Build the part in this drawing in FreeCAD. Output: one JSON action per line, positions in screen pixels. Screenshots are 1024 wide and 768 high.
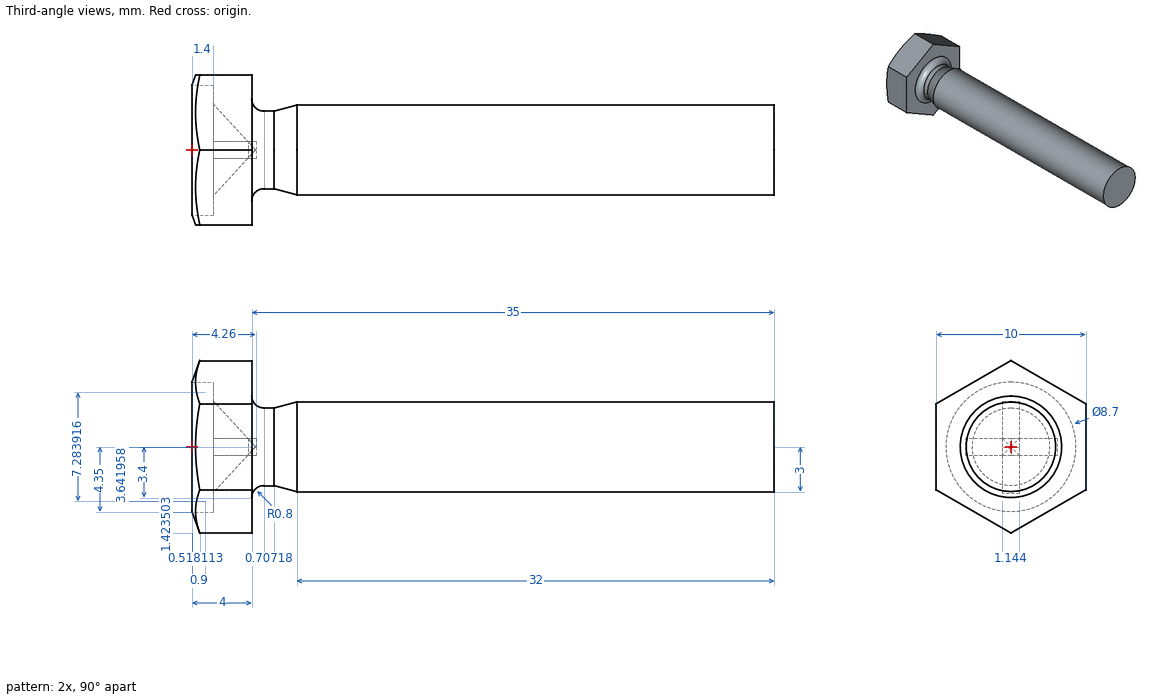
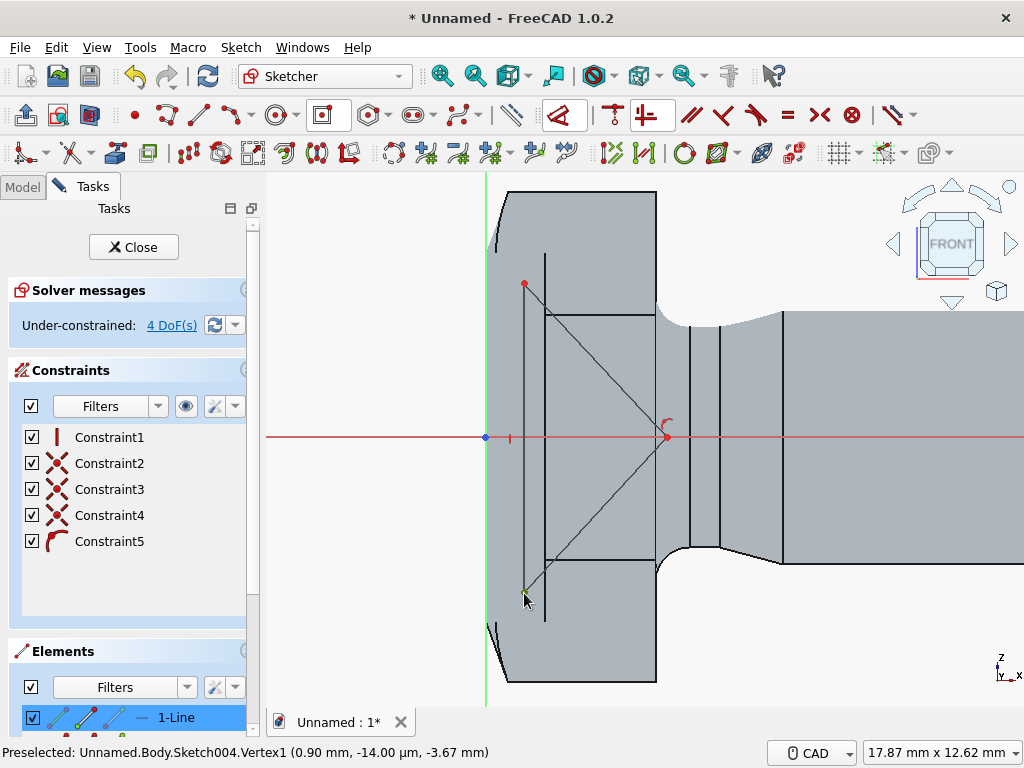
{"action": "left_click", "coordinate": [582, 116]}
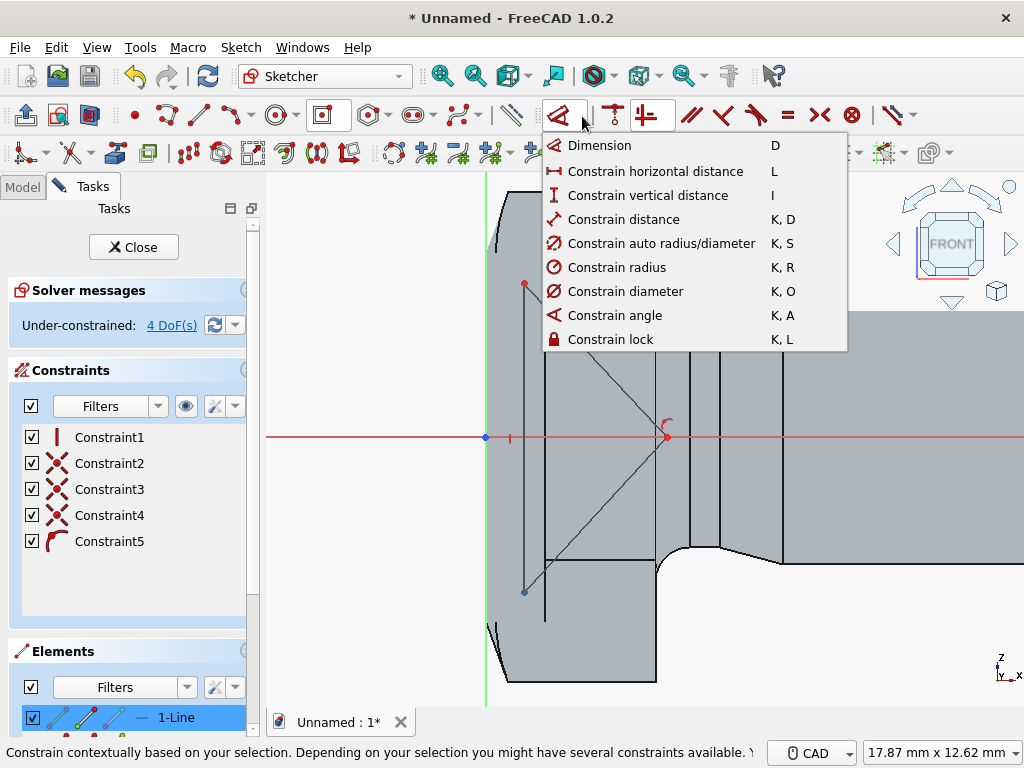
{"action": "left_click", "coordinate": [695, 171]}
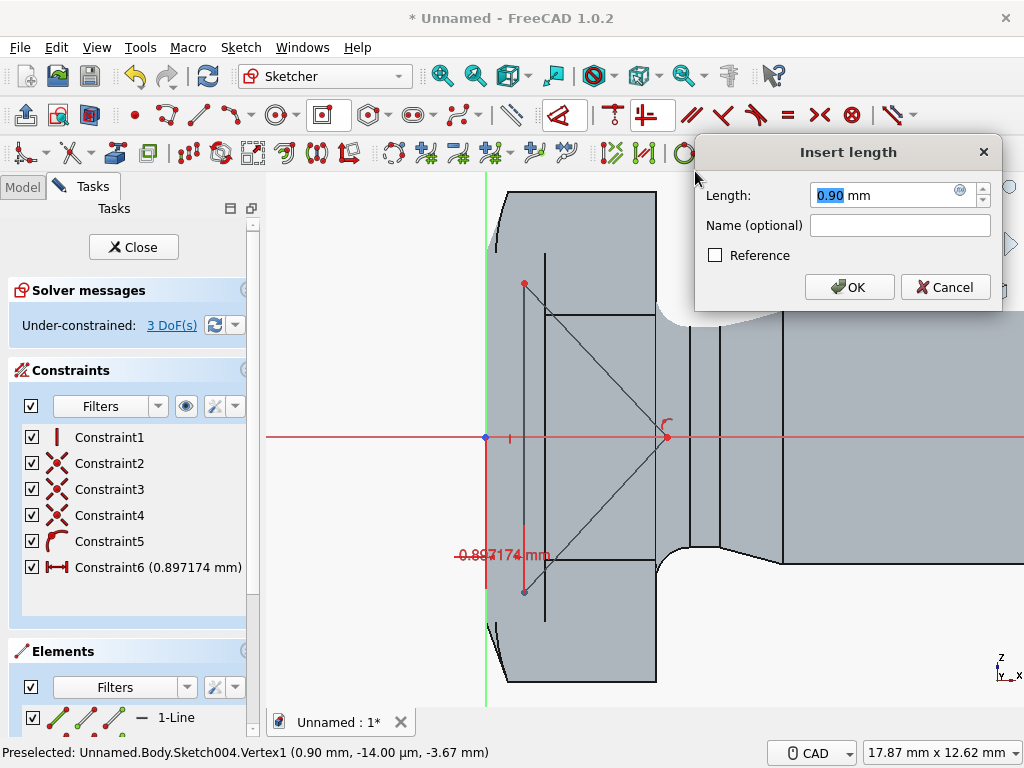
{"action": "type", "text": "0.9"}
{"action": "key", "text": "Return"}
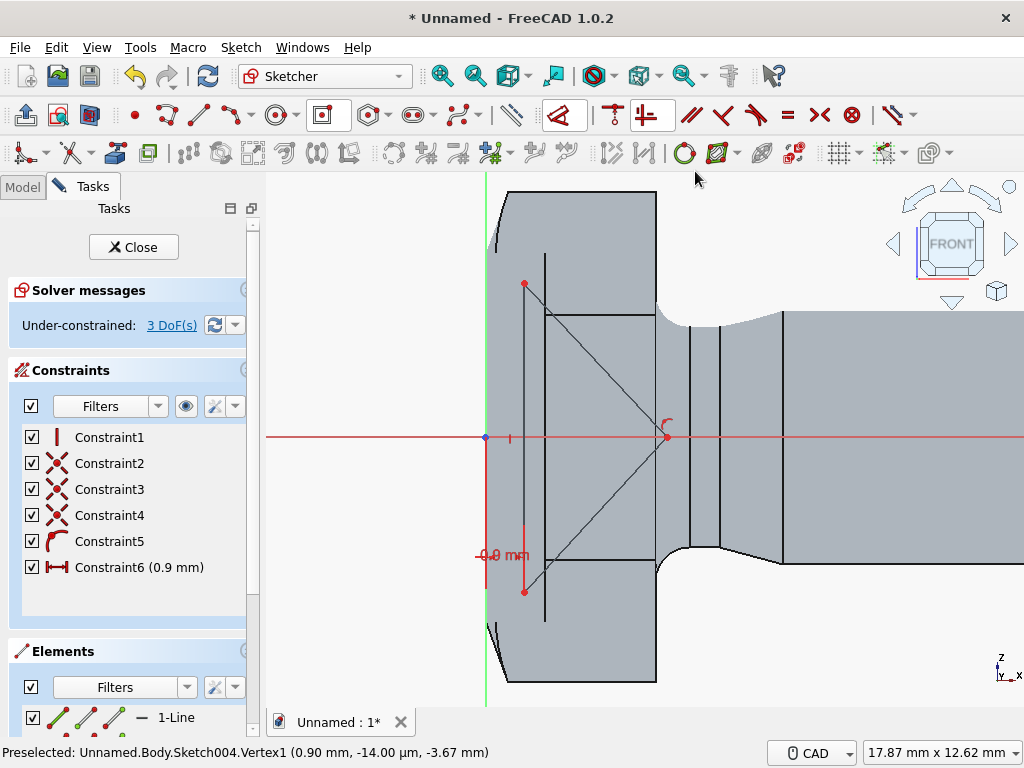
{"action": "left_click", "coordinate": [667, 437]}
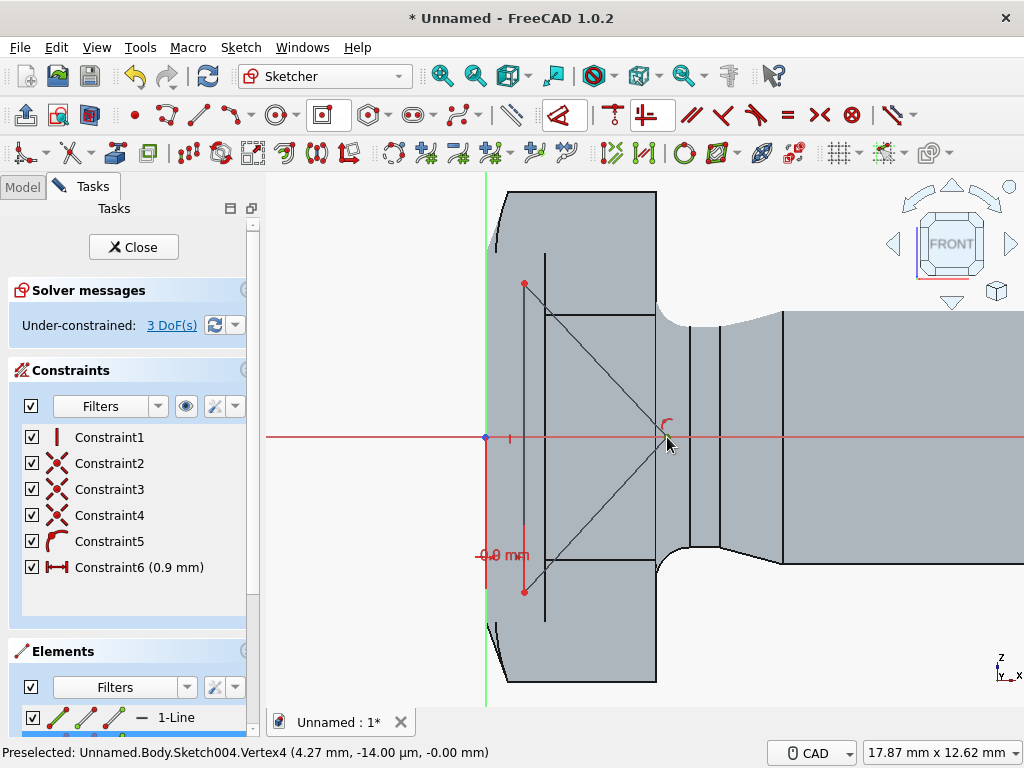
{"action": "key", "text": "l"}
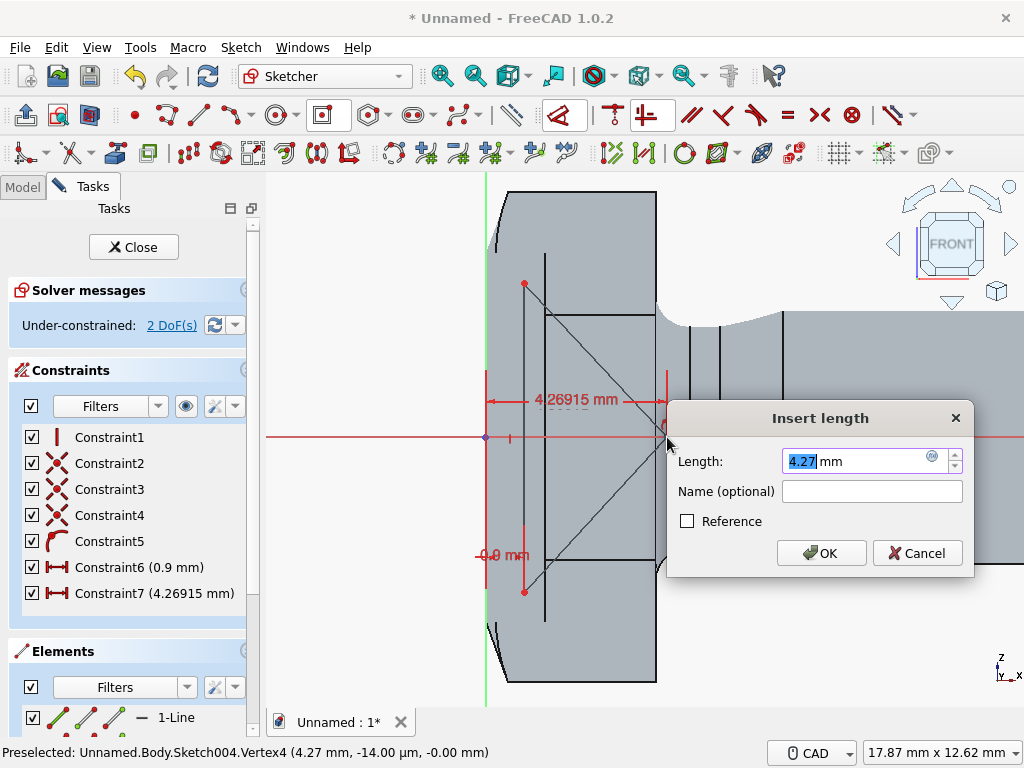
{"action": "type", "text": "4.26"}
{"action": "key", "text": "Return"}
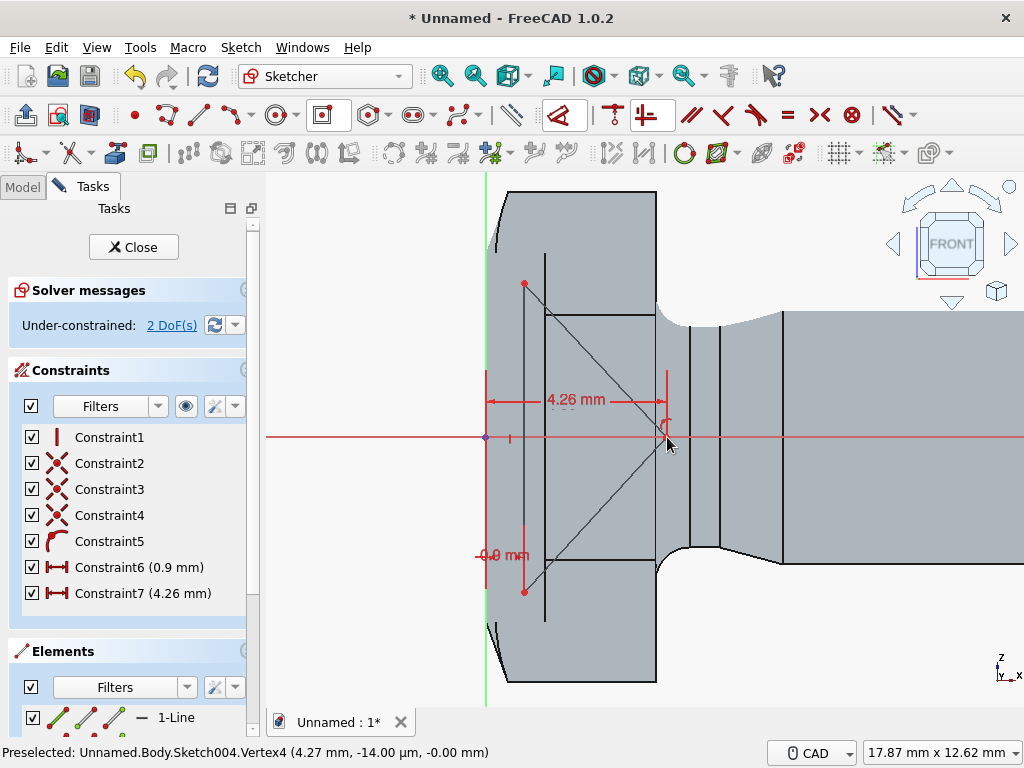
{"action": "left_click", "coordinate": [524, 500]}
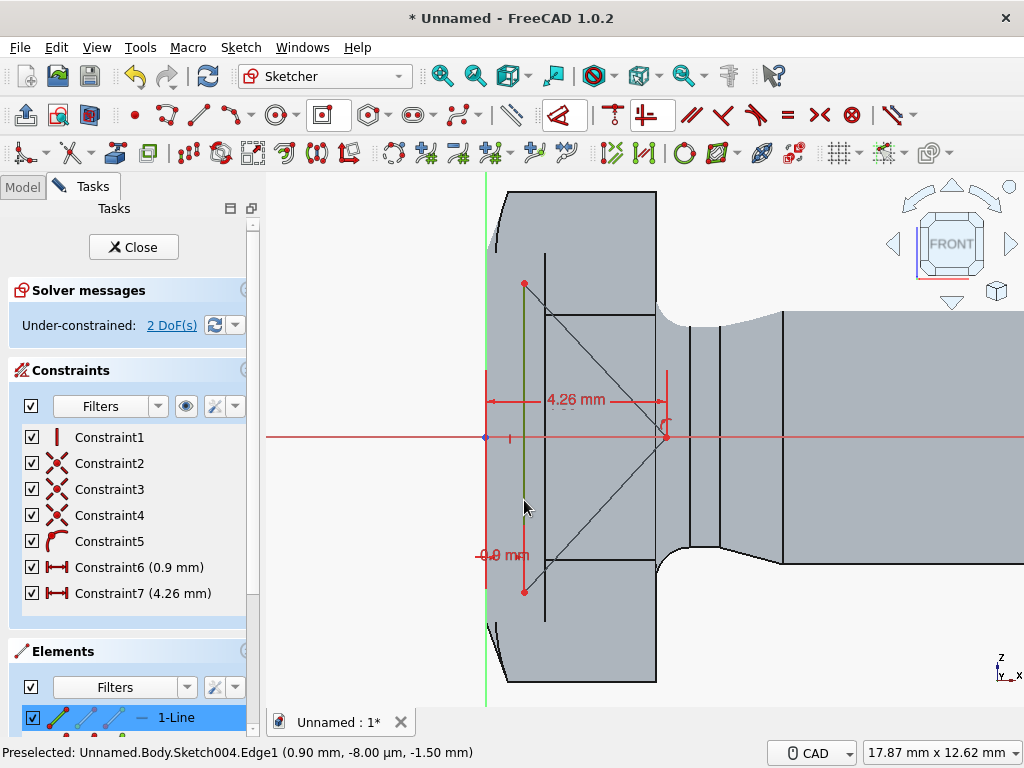
{"action": "key", "text": "i"}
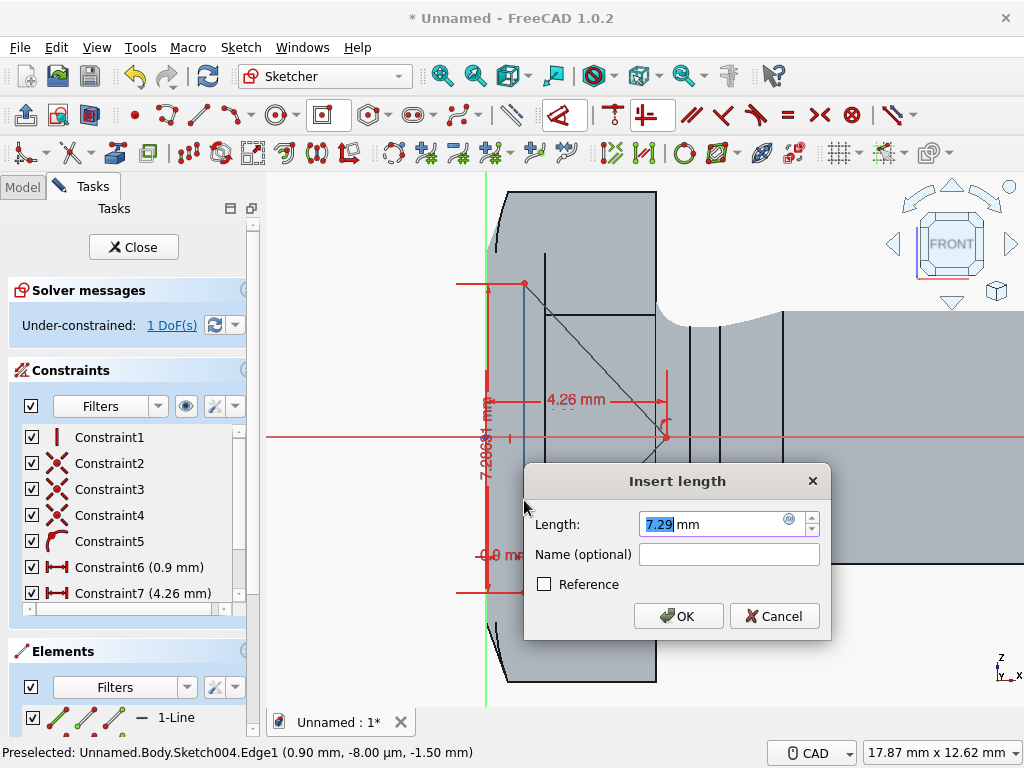
{"action": "type", "text": "7.283916"}
{"action": "key", "text": "Return"}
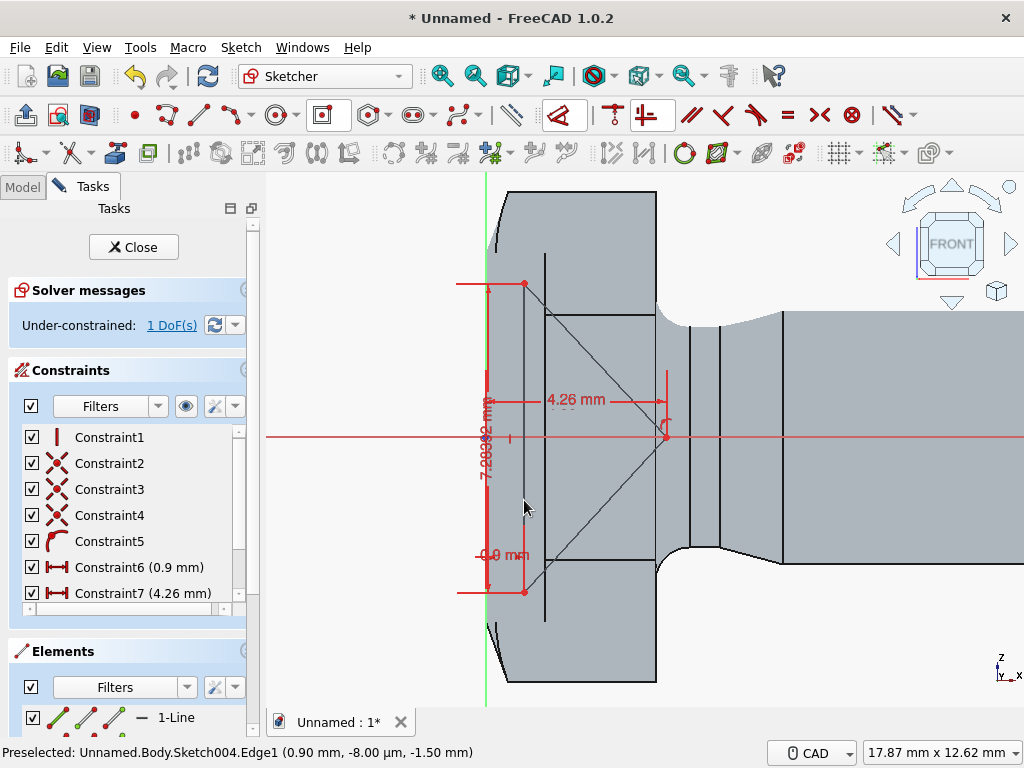
{"action": "left_click", "coordinate": [524, 593]}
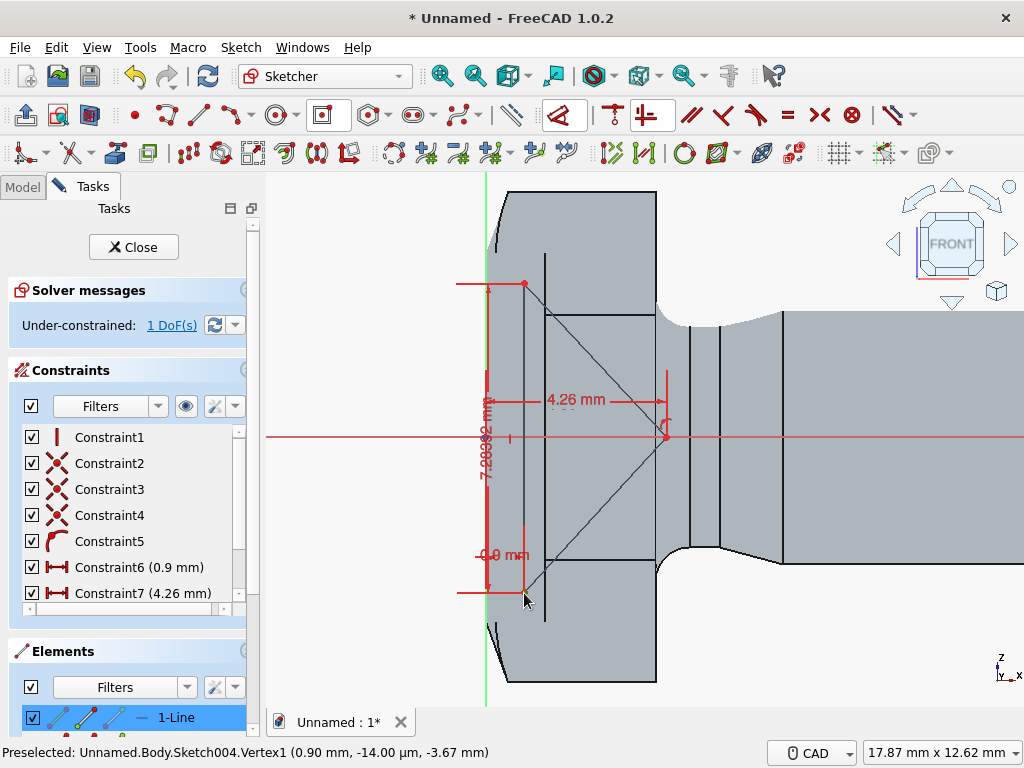
{"action": "left_click", "coordinate": [582, 116]}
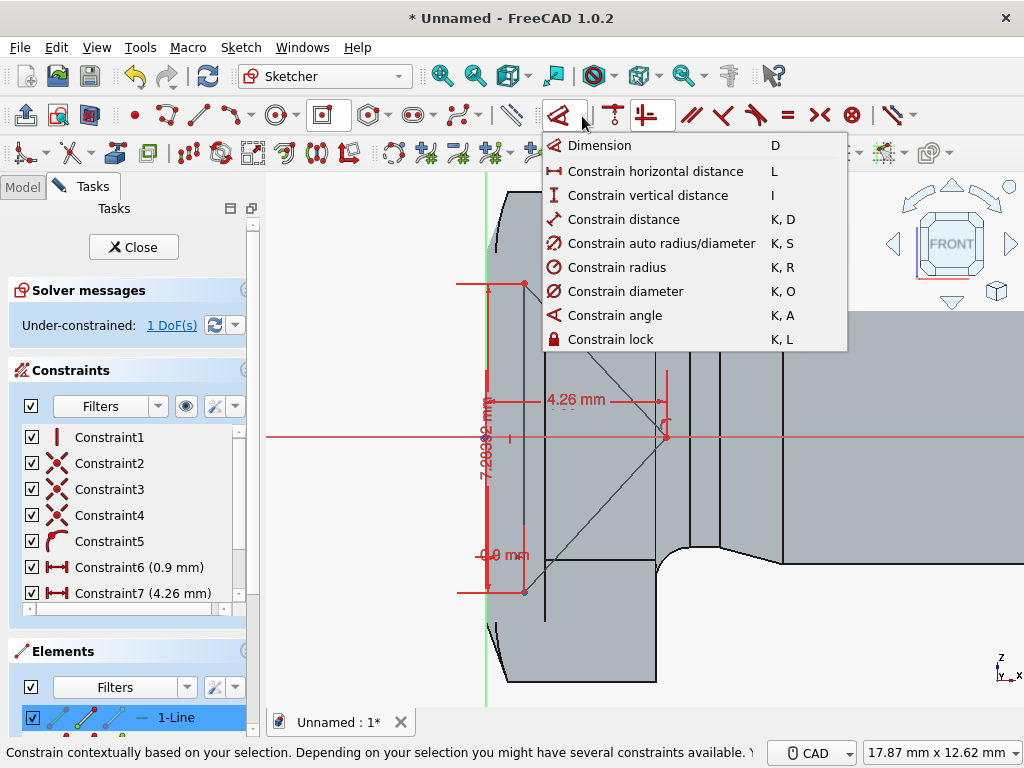
{"action": "left_click", "coordinate": [695, 195]}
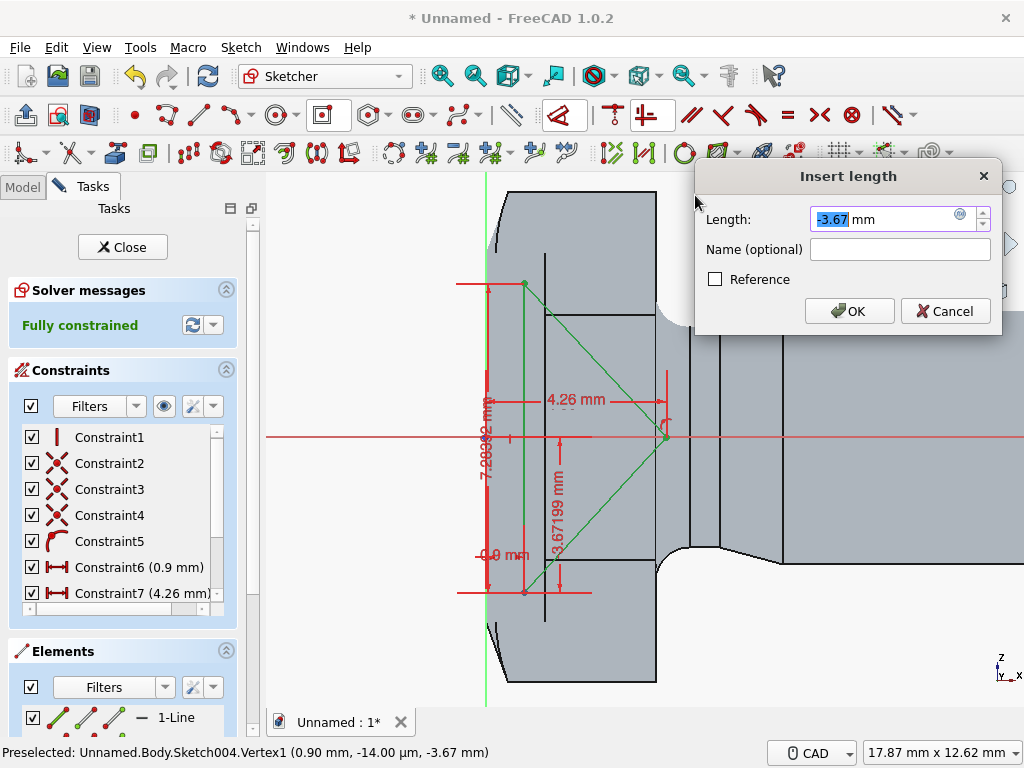
{"action": "type", "text": "-3.641958"}
{"action": "key", "text": "Return"}